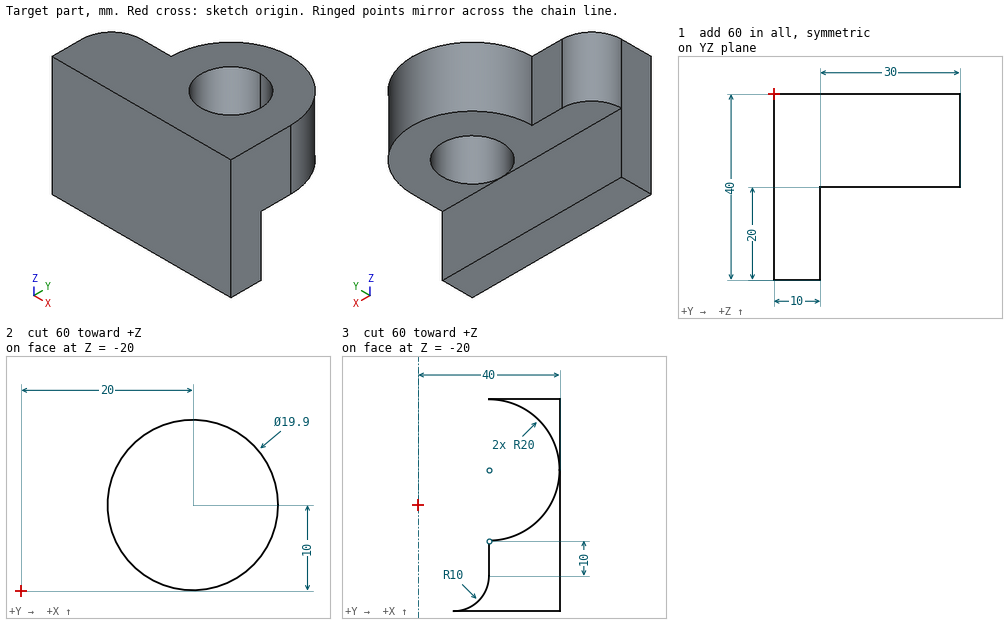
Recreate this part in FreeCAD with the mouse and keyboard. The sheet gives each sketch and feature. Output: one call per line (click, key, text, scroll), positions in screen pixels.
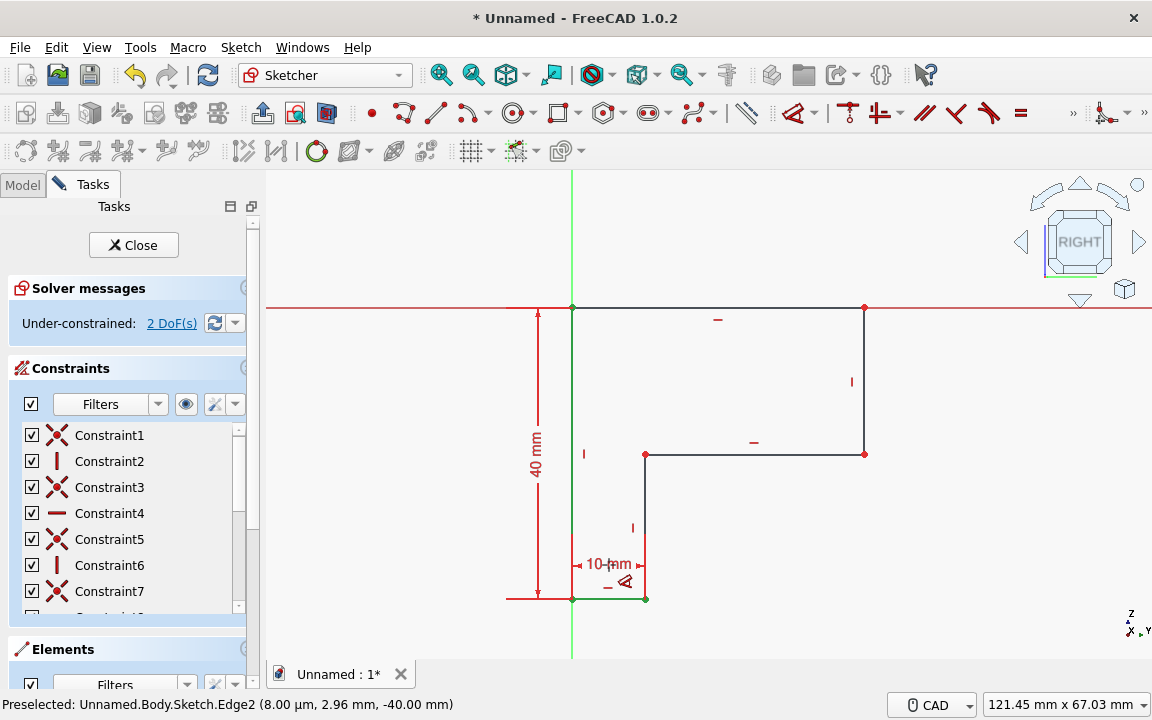
click(645, 556)
click(611, 527)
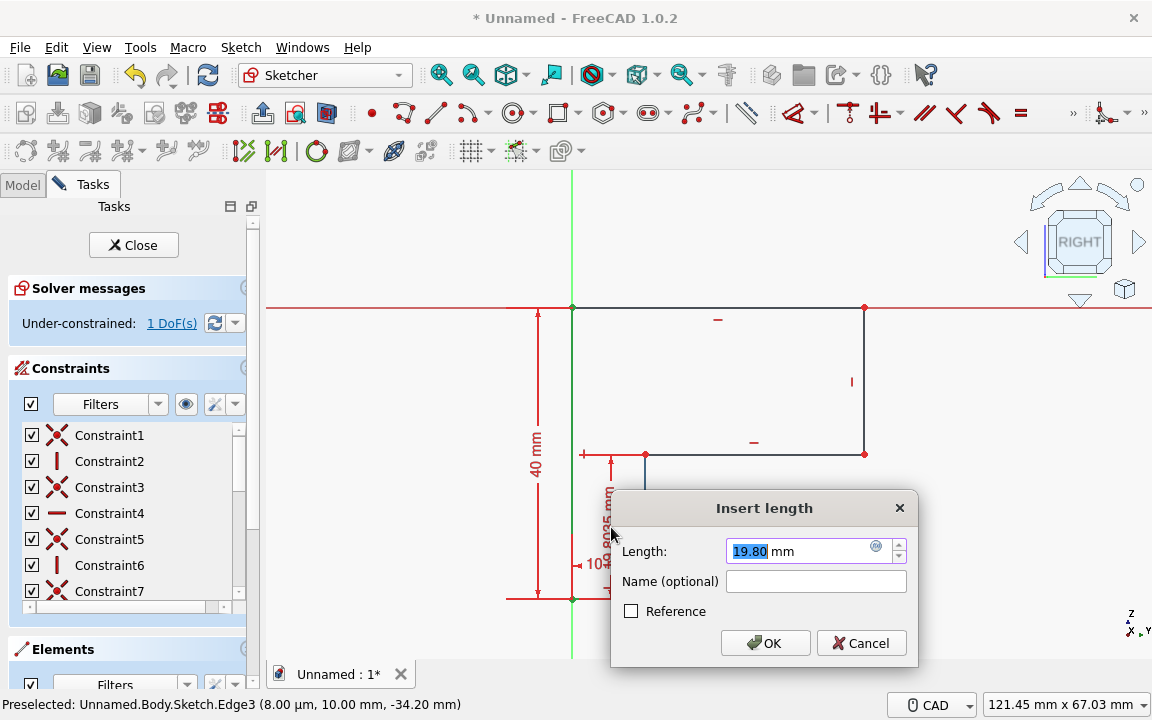
text(20)
key(Return)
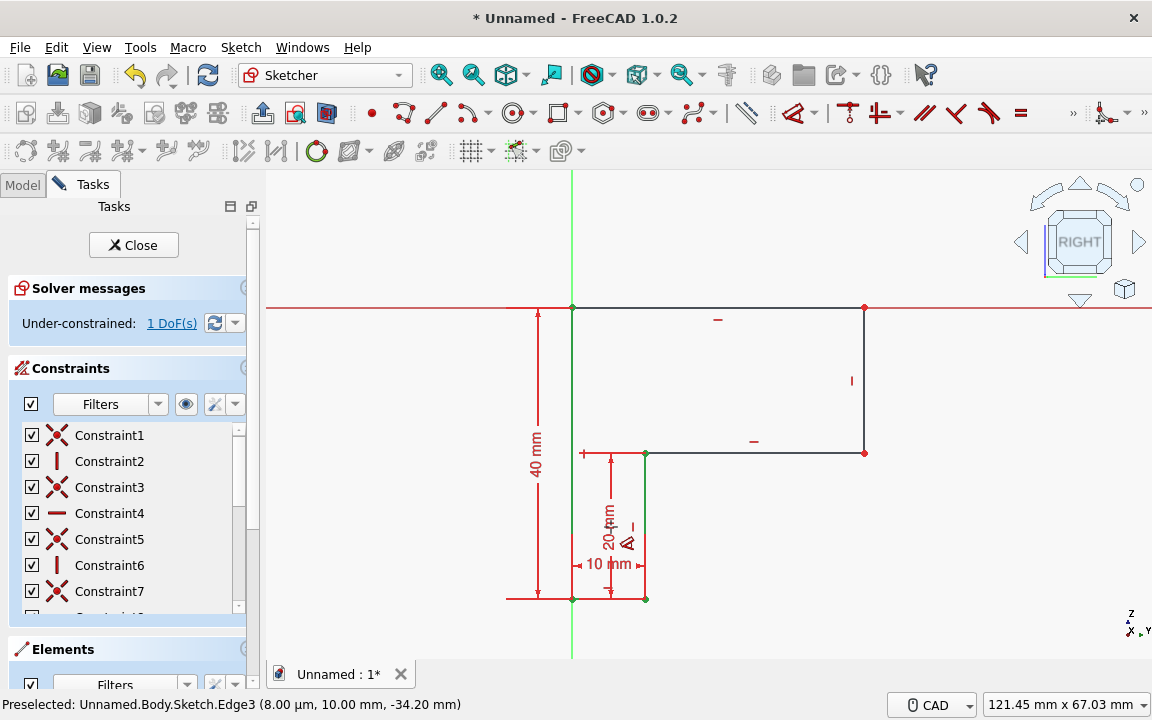
click(711, 453)
click(755, 487)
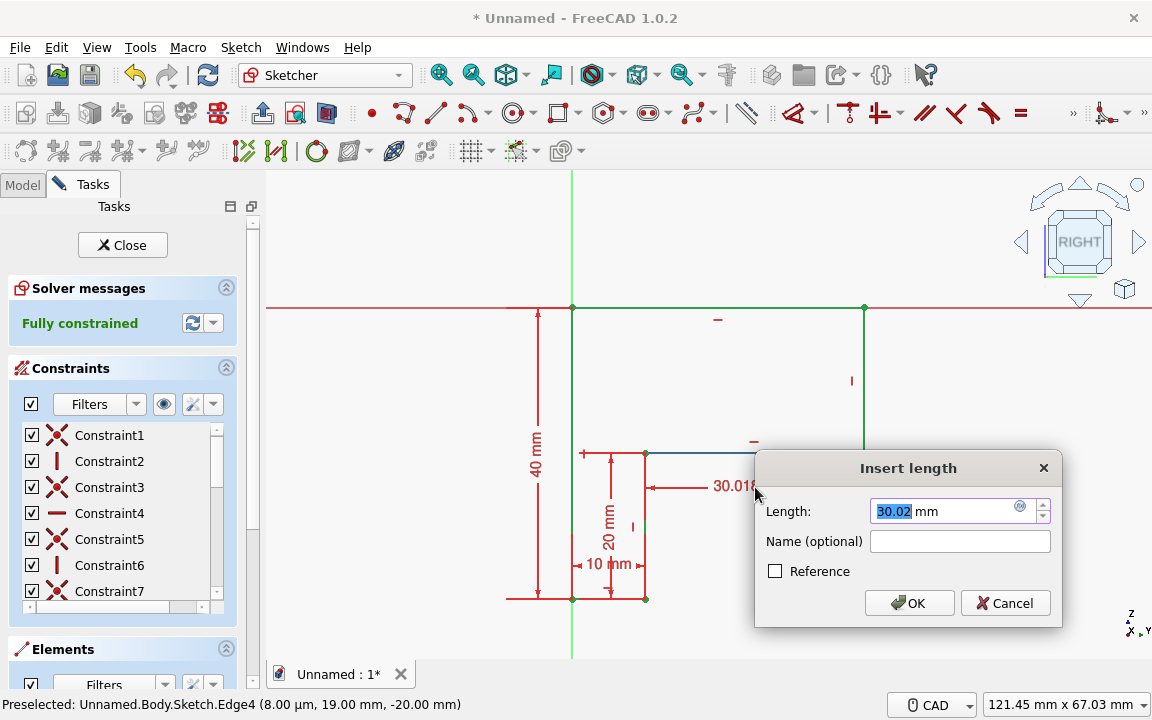
text(30)
key(Return)
key(Escape)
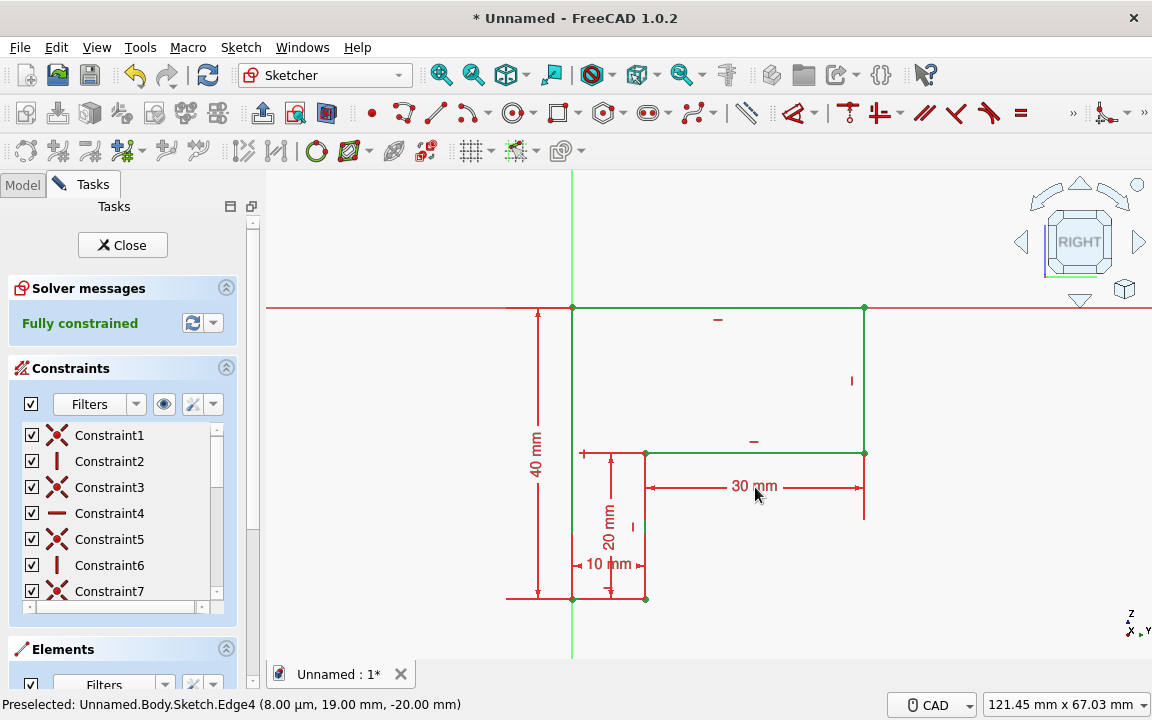
click(123, 245)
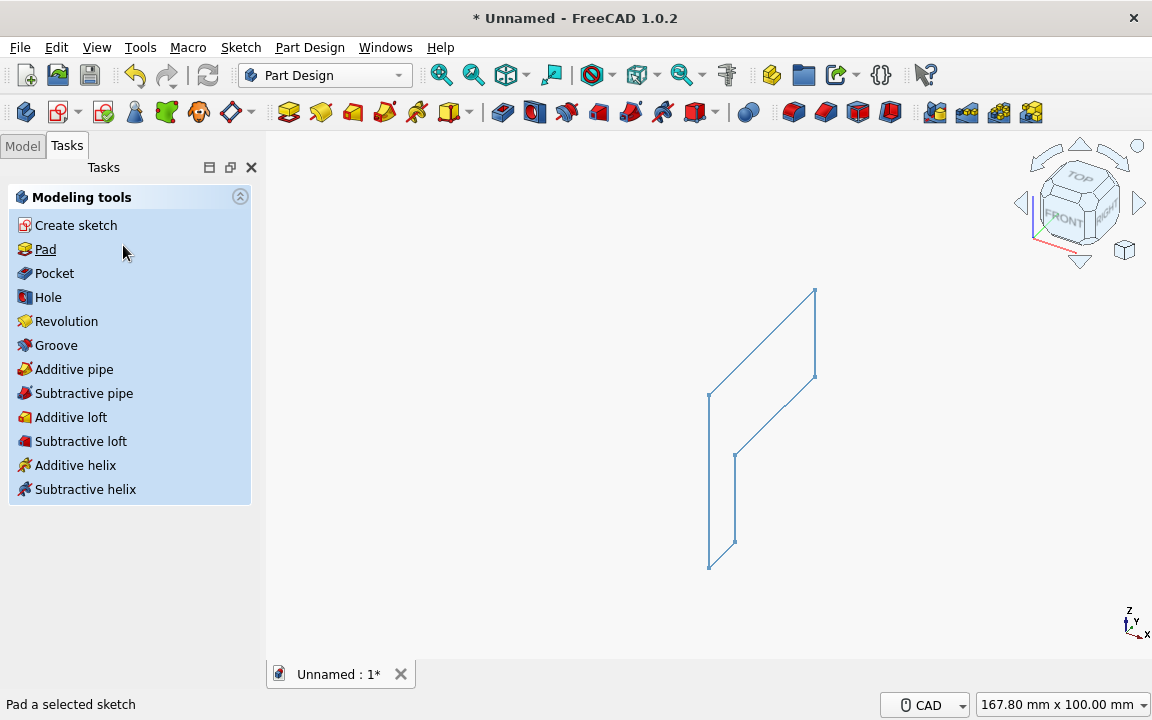
click(290, 112)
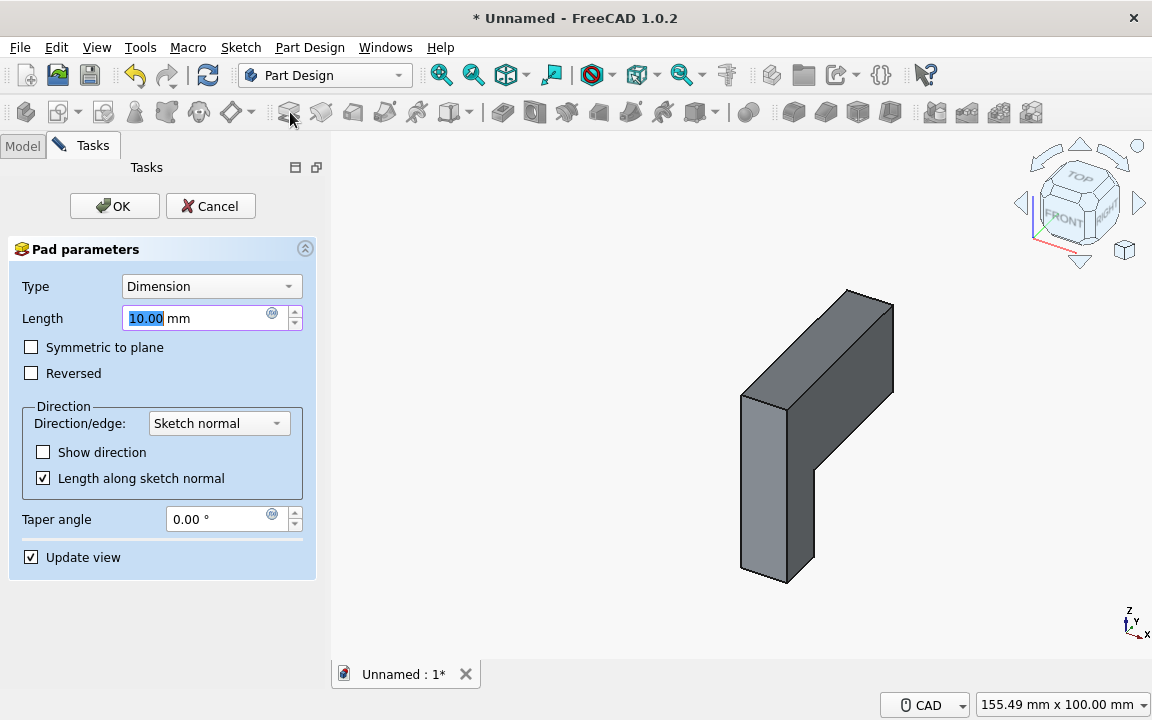
text(60)
key(Tab)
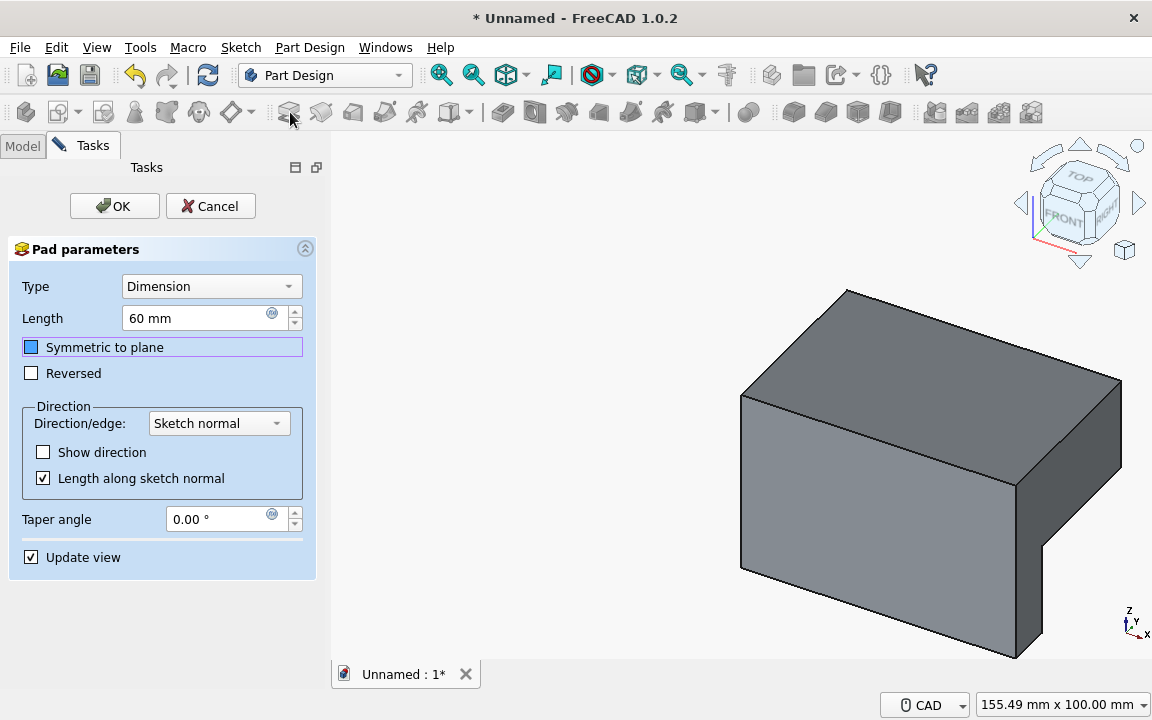
click(30, 347)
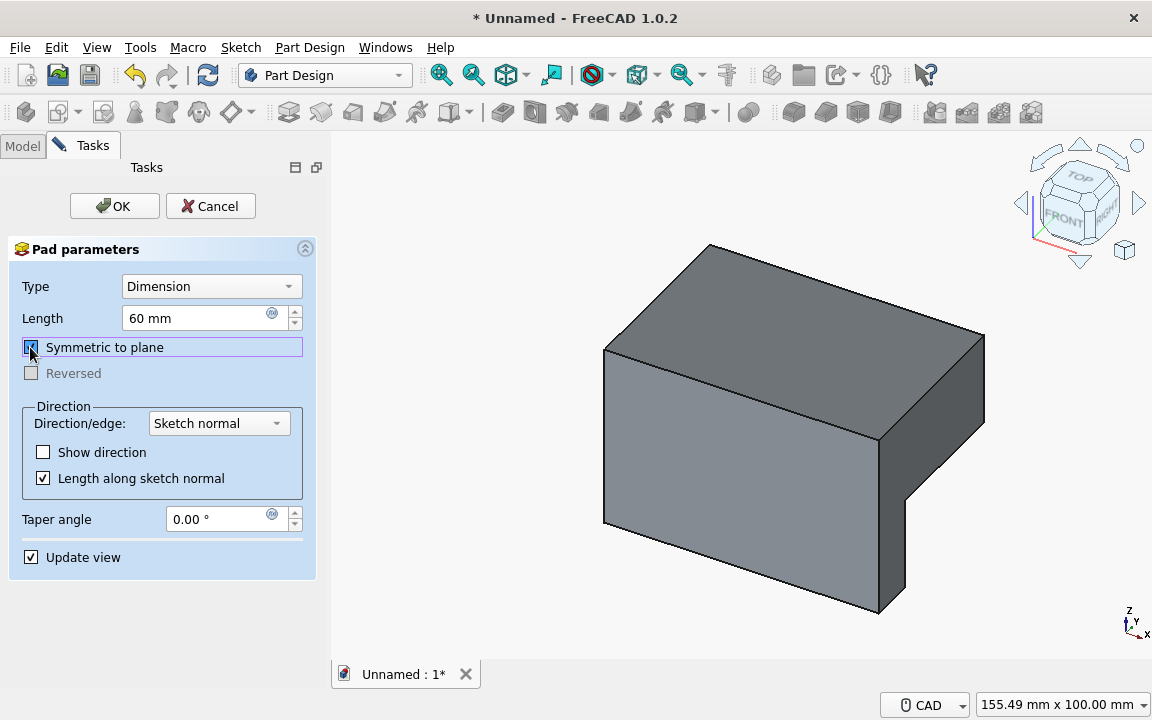
click(115, 206)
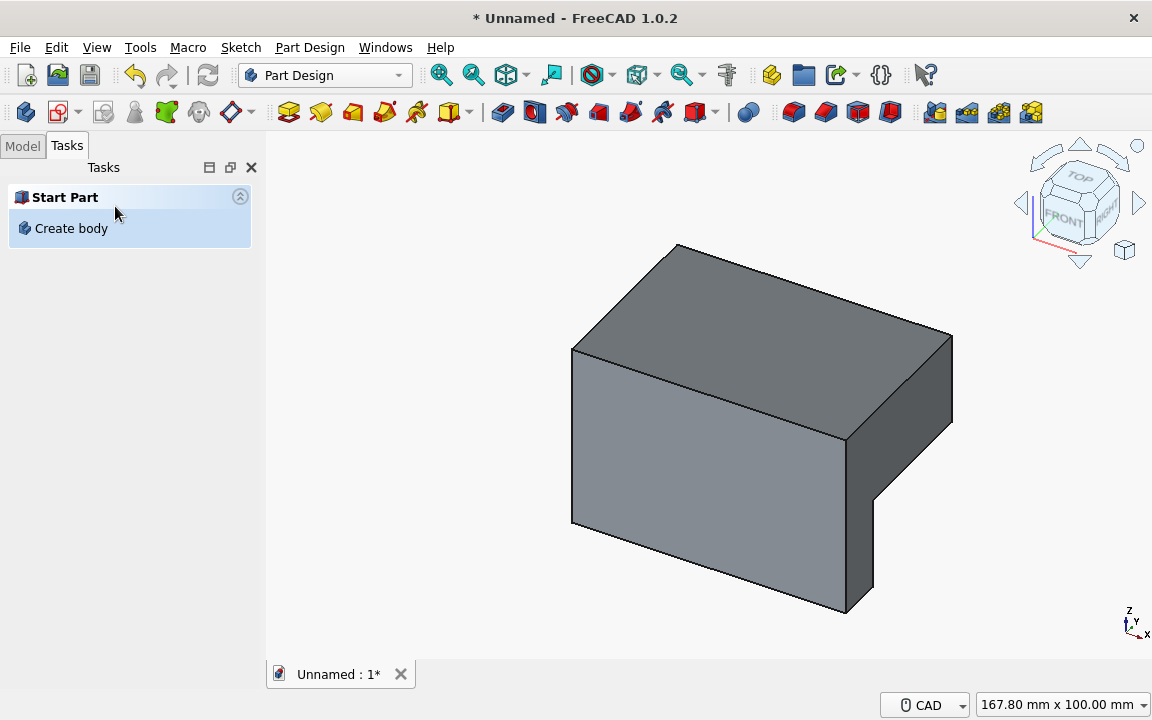
key(5)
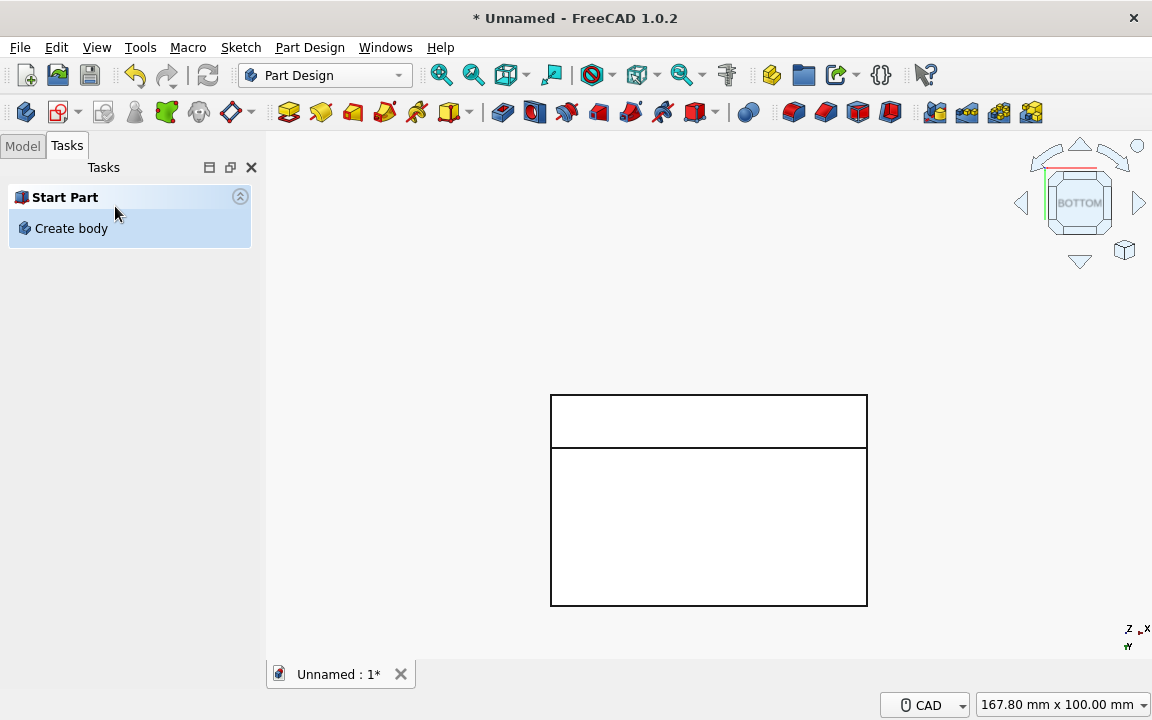
click(442, 76)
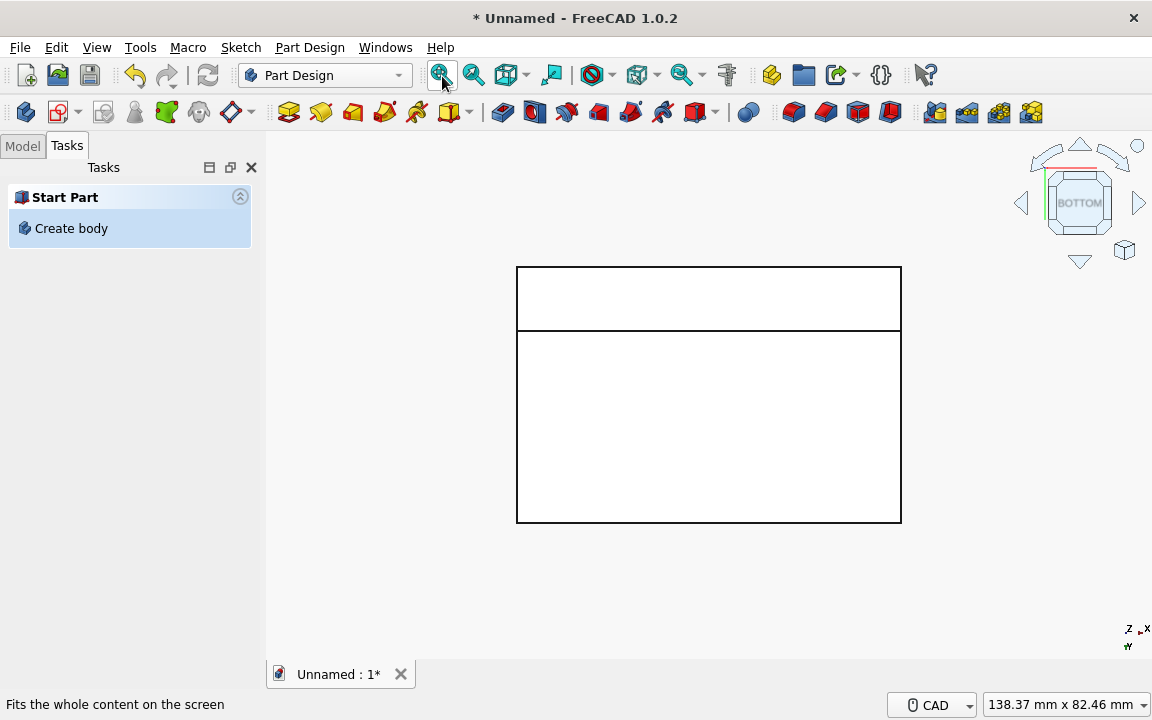
click(764, 426)